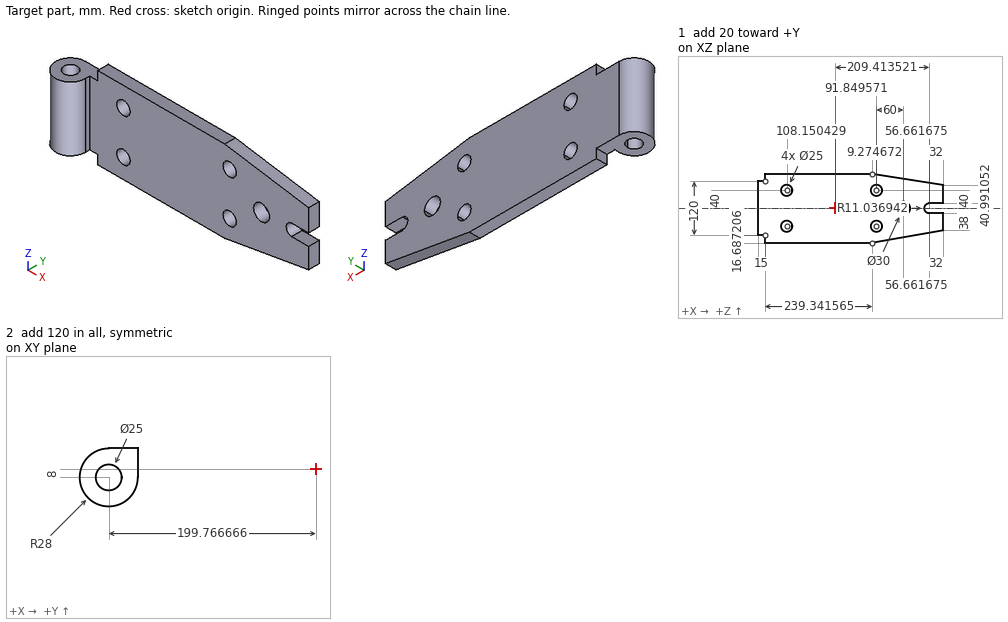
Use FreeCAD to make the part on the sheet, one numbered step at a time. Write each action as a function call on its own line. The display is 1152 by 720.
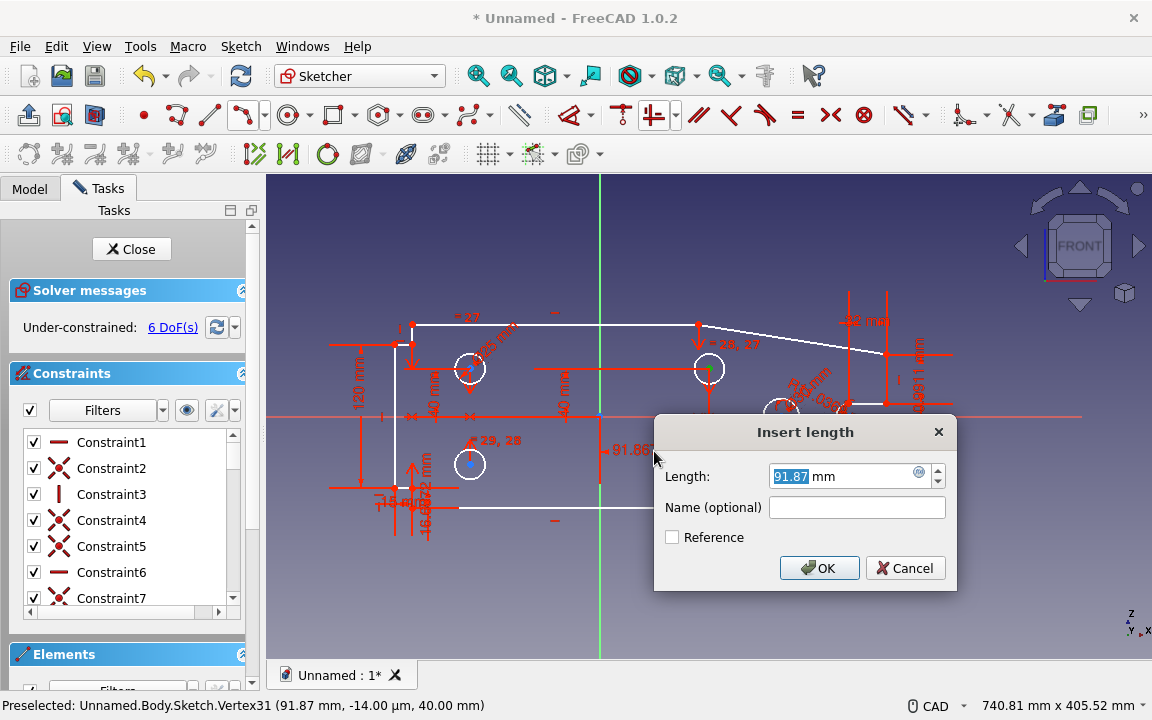
text(91.849571)
key(Return)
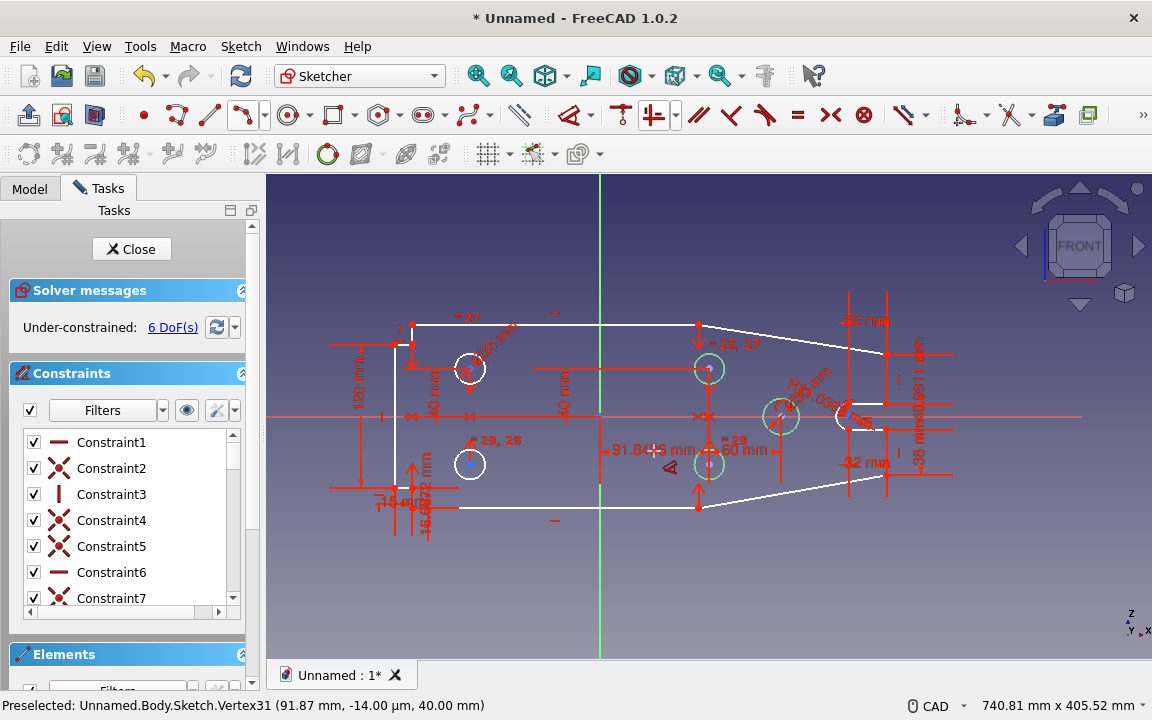
scroll(699, 325, up, 7)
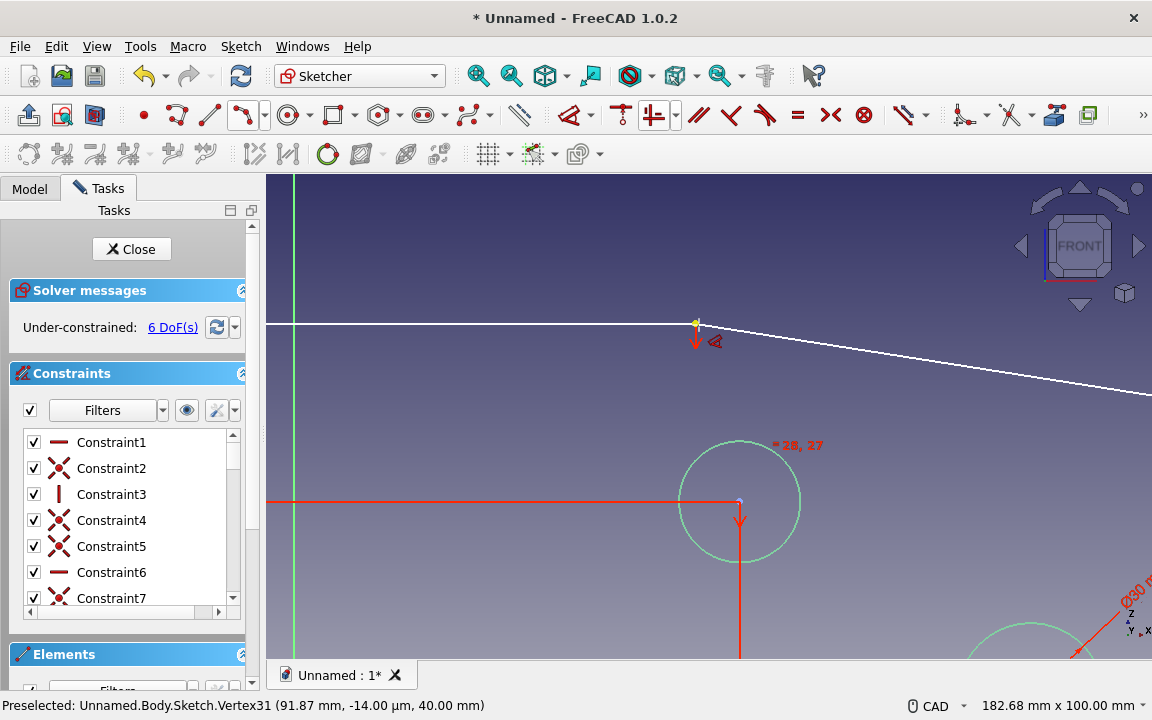
click(696, 324)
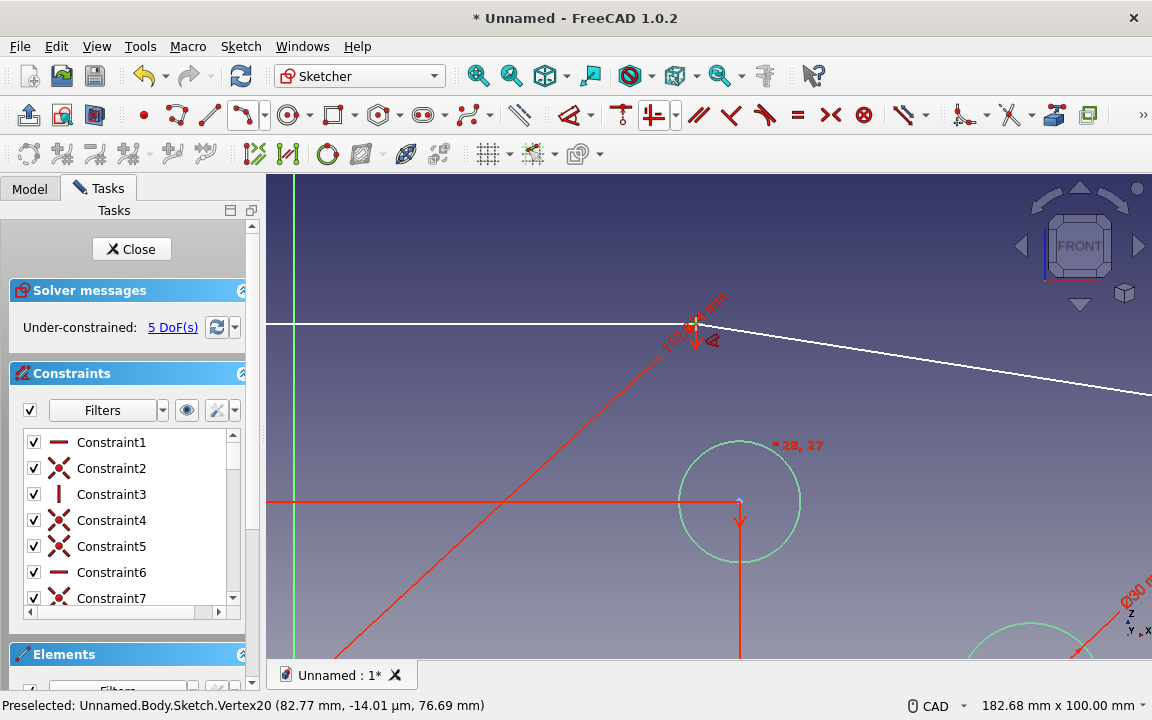
click(740, 502)
click(718, 290)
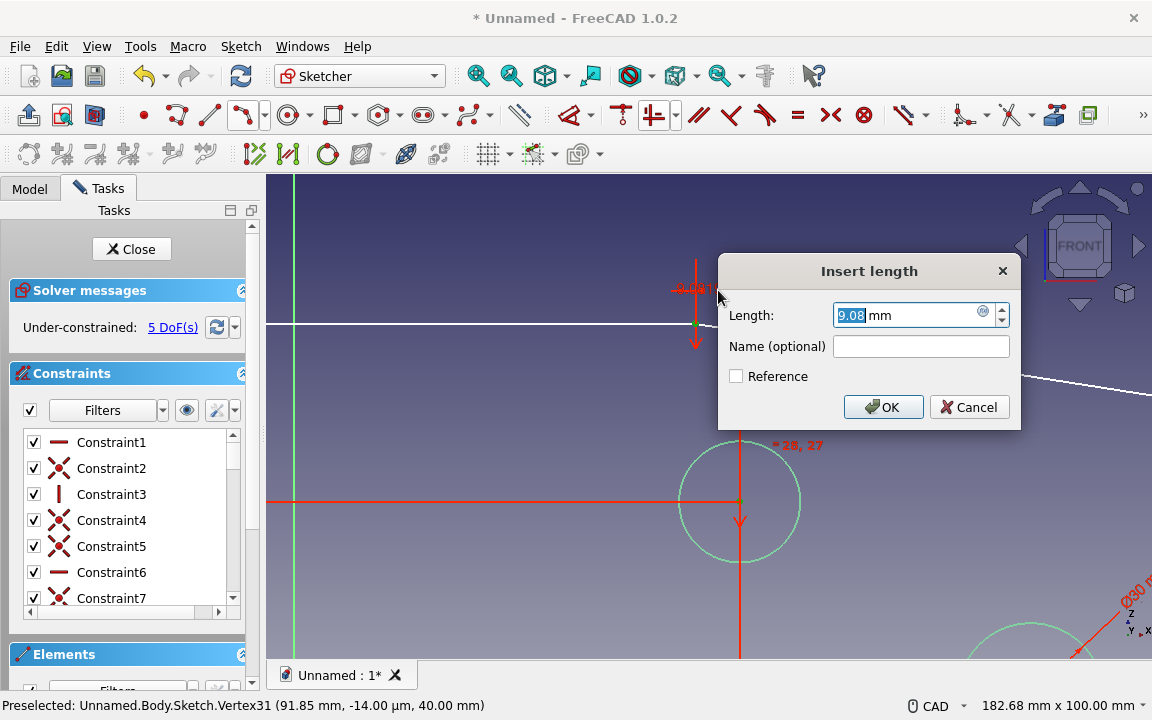
text(9.274672)
key(Return)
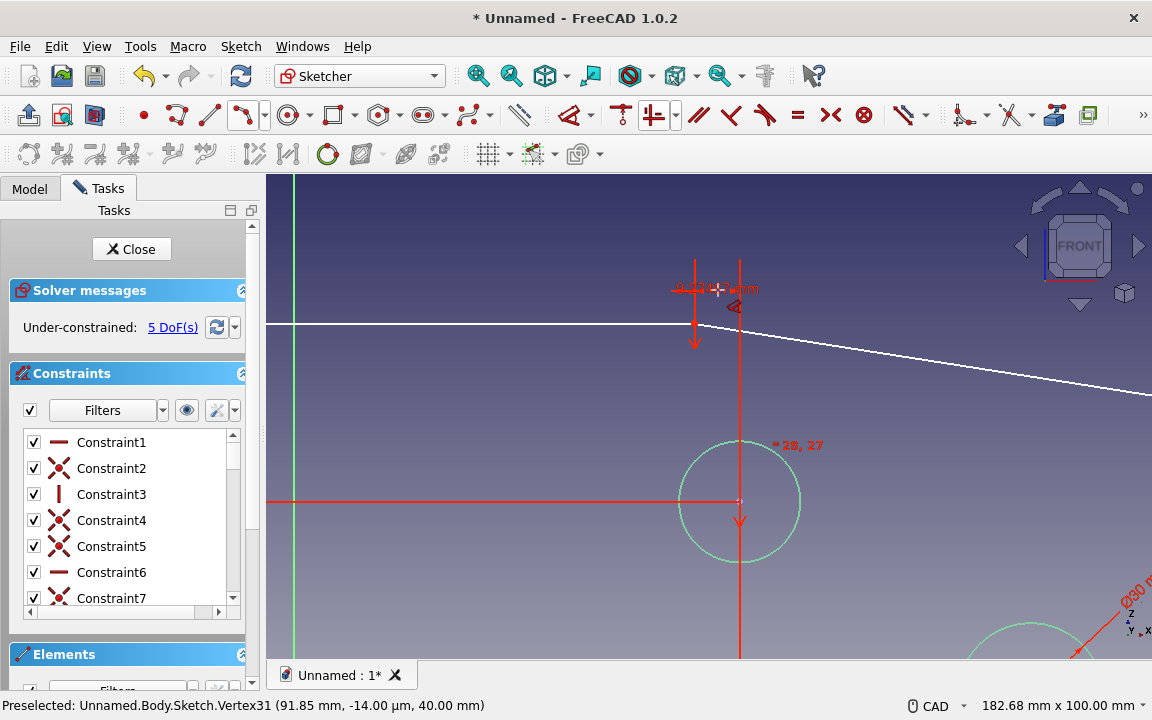
scroll(699, 325, down, 7)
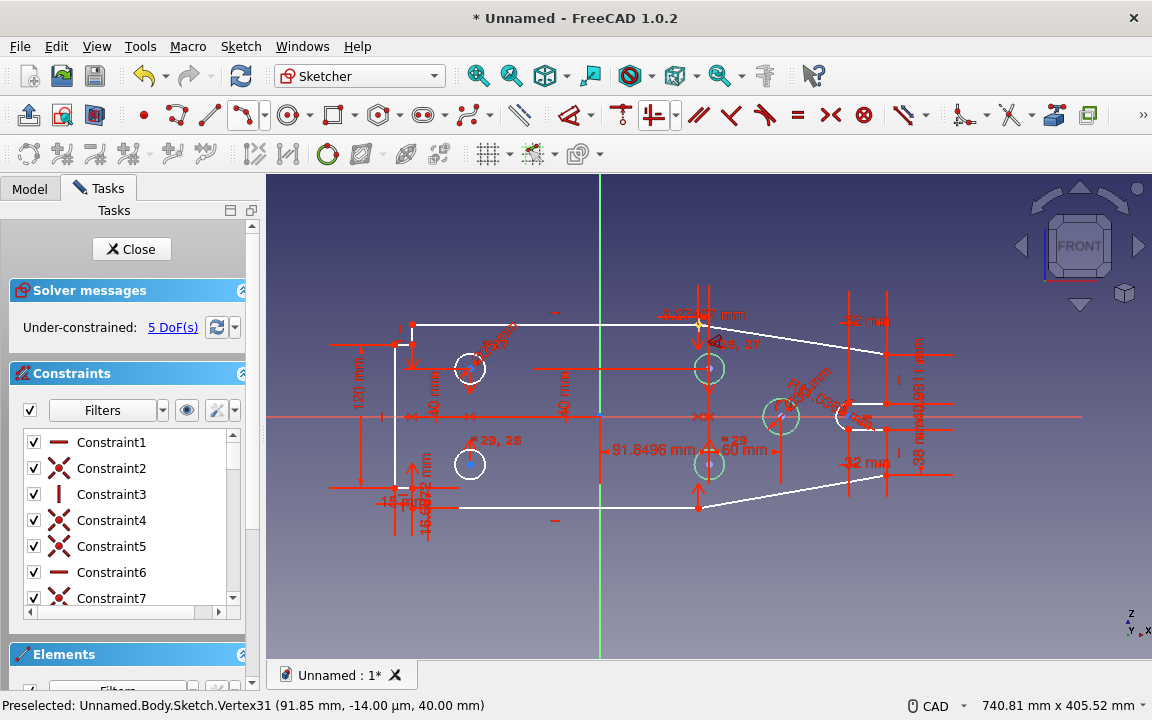
click(613, 508)
click(555, 542)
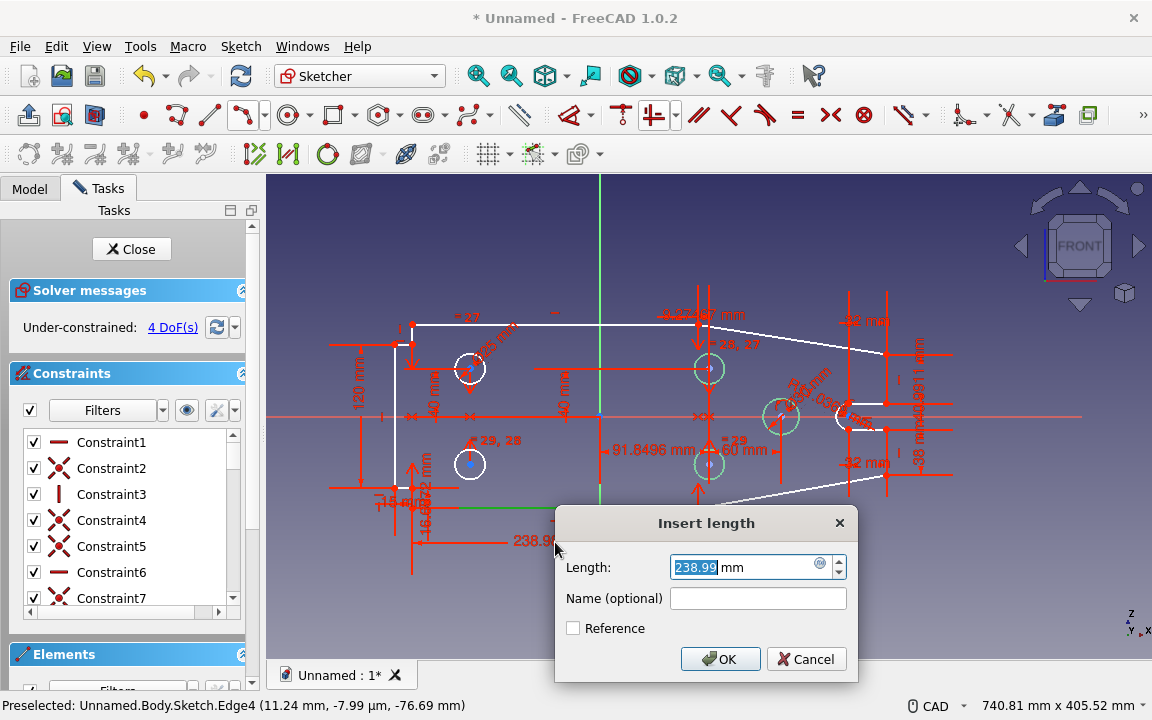
text(239.341565)
key(Return)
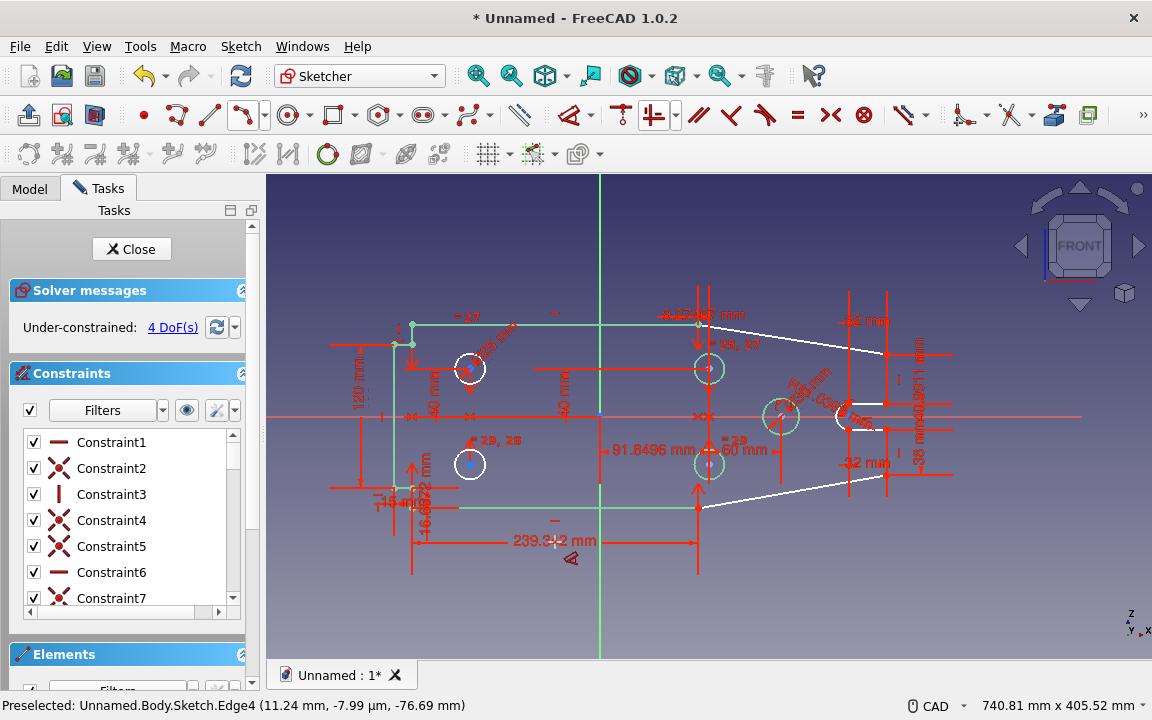
click(470, 369)
click(535, 451)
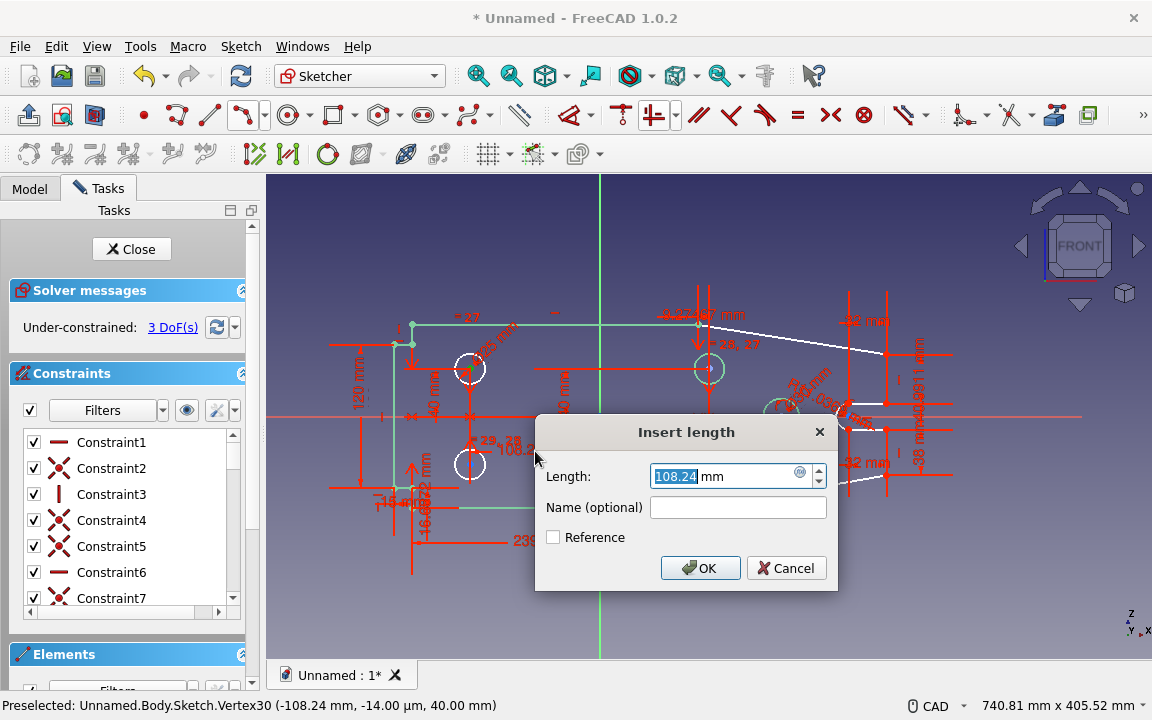
text(108.150429)
key(Return)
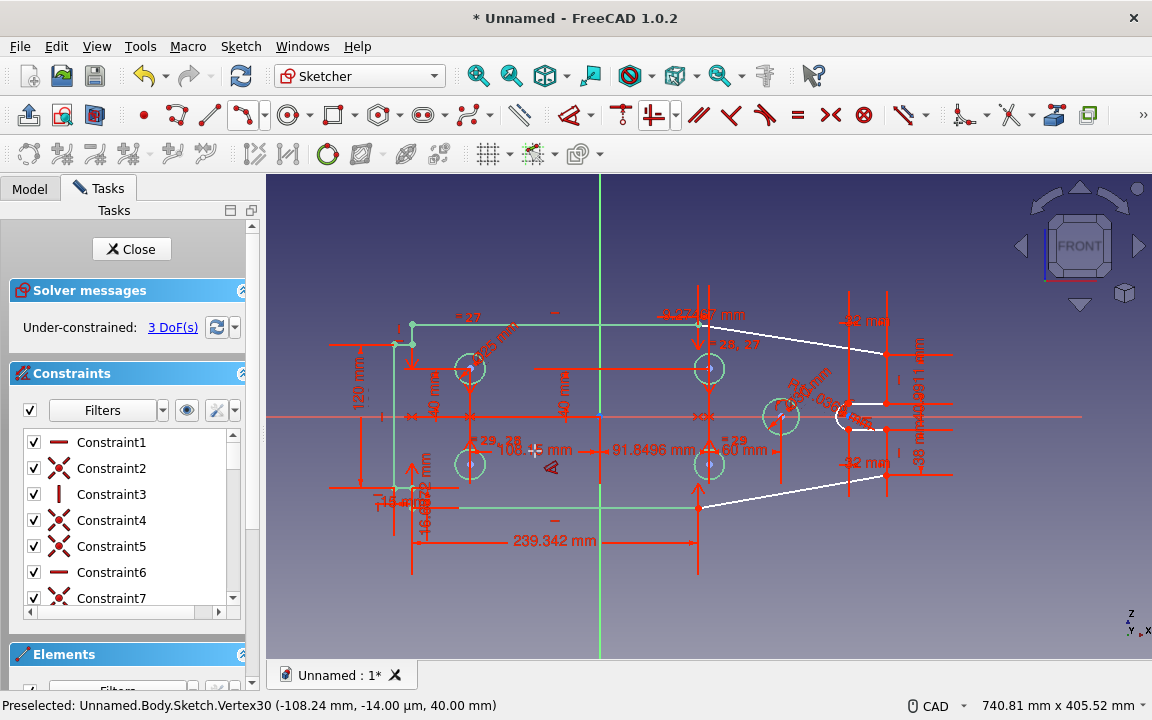
click(849, 404)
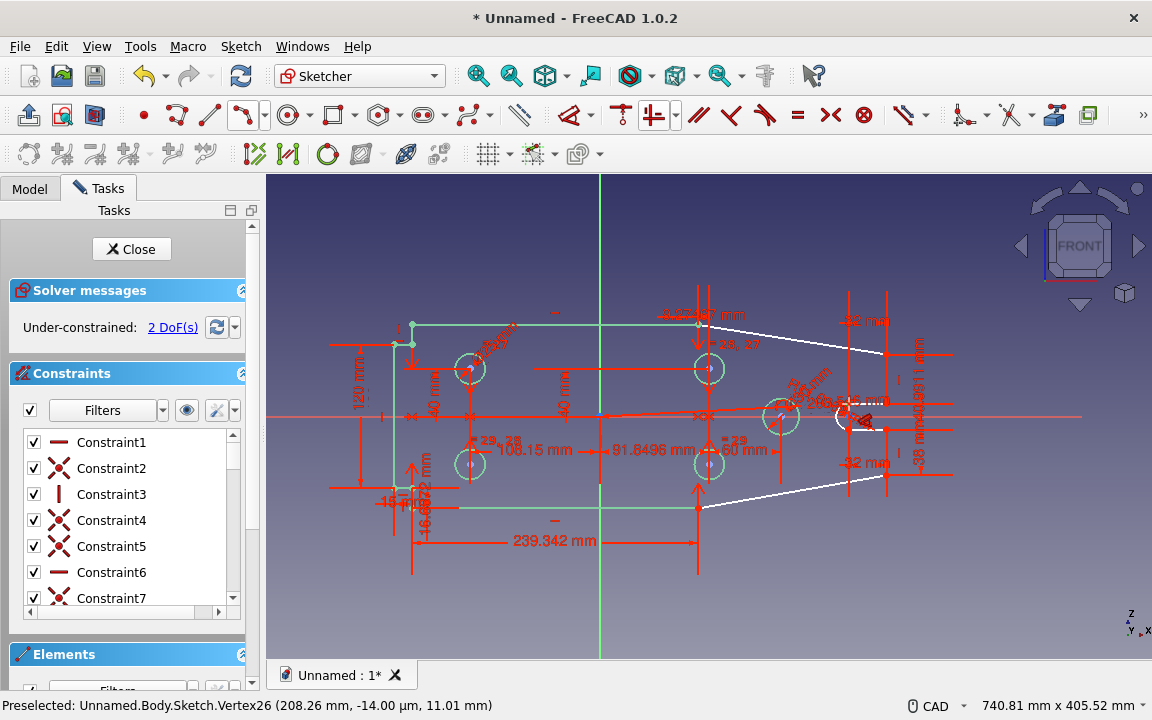
click(781, 417)
click(791, 475)